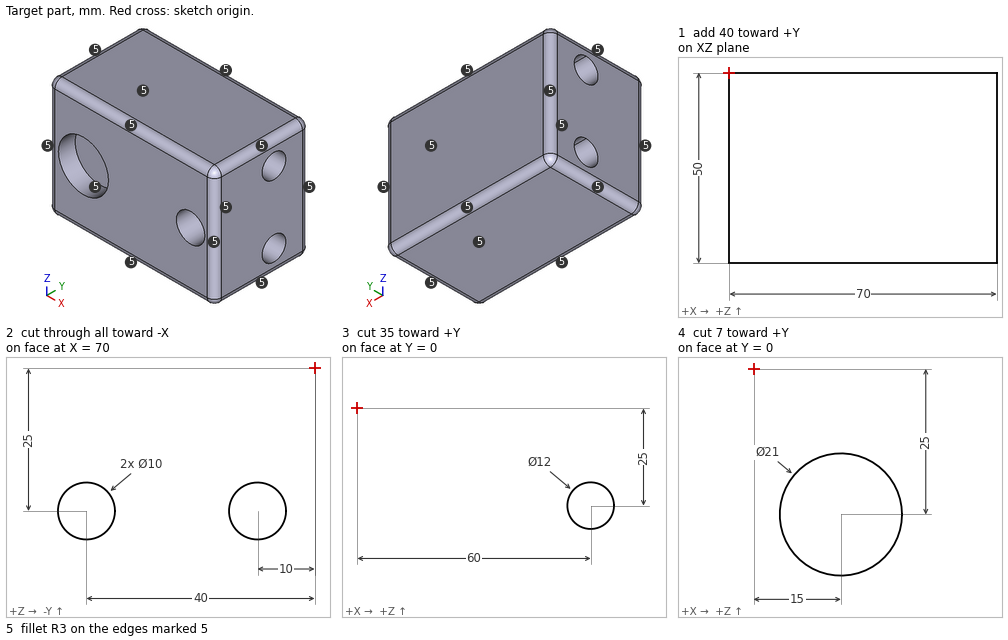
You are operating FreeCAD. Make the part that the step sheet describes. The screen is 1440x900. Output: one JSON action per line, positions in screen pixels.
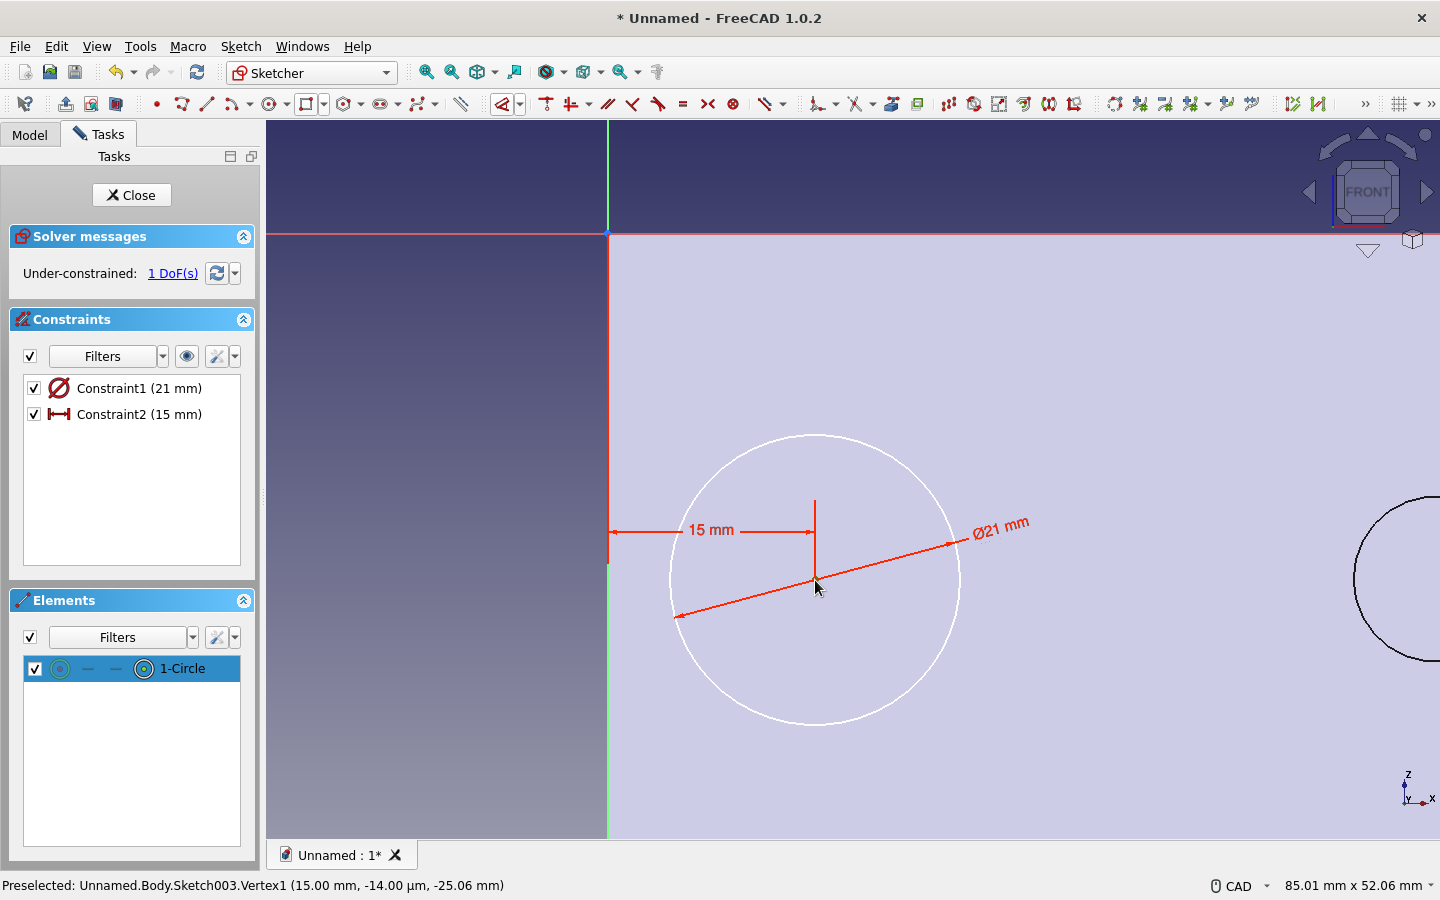
{"action": "key", "text": "i"}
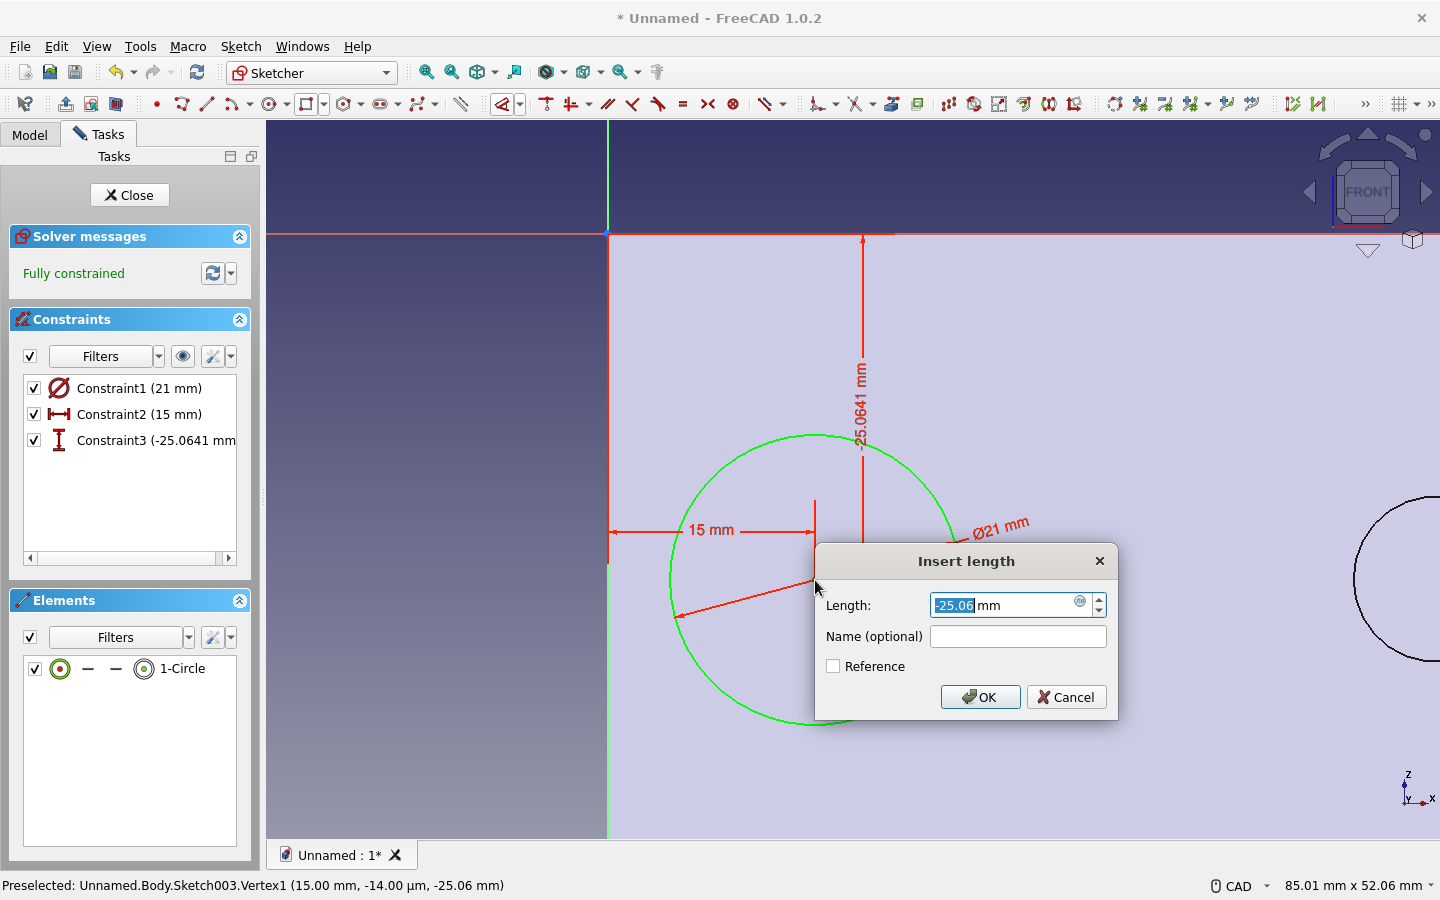
{"action": "type", "text": "-25"}
{"action": "key", "text": "Return"}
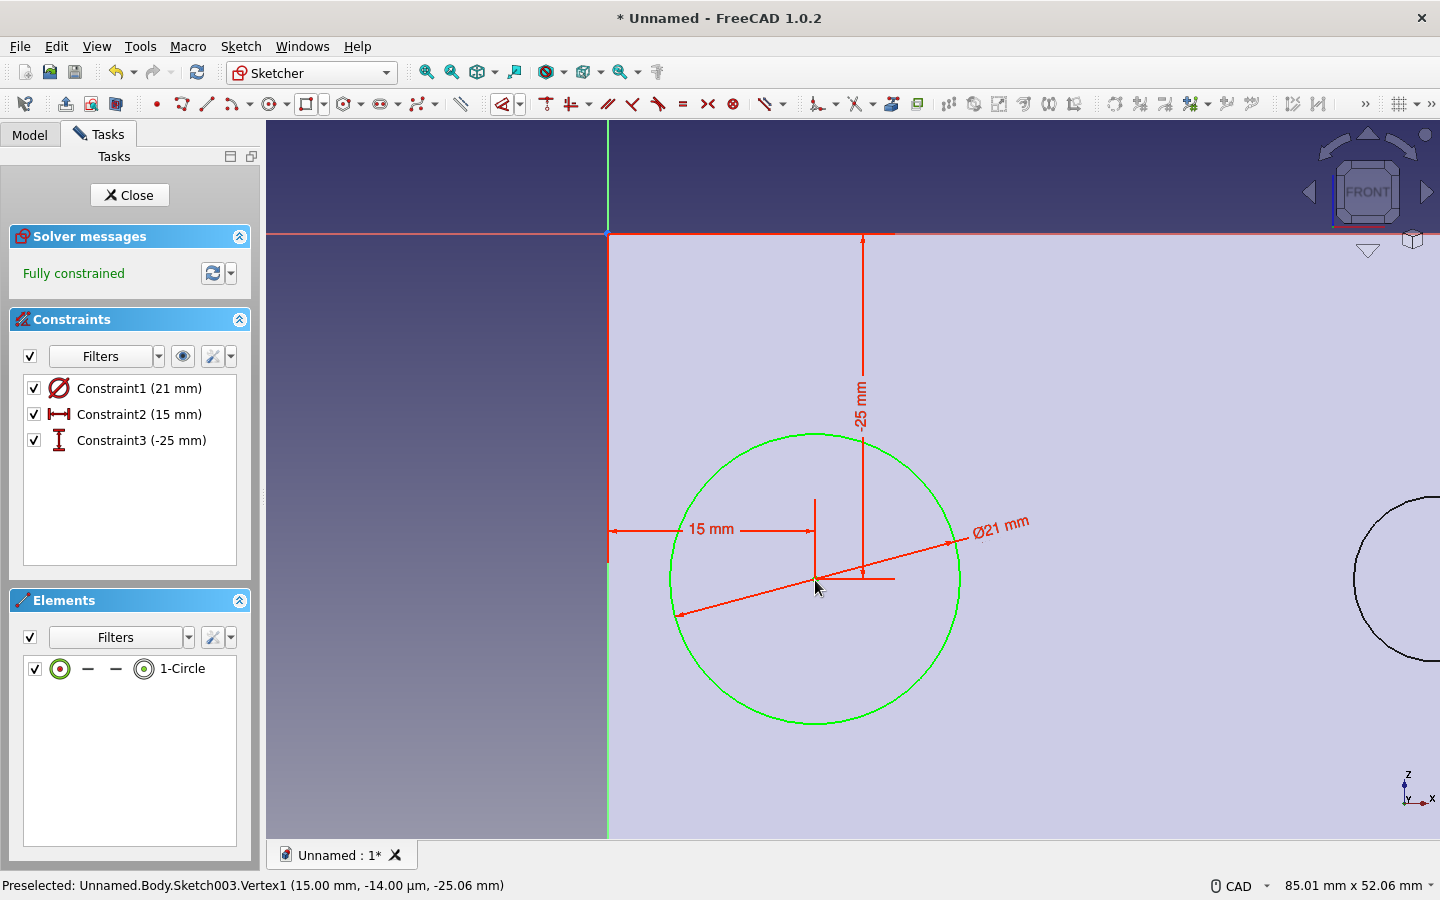
{"action": "left_click", "coordinate": [130, 195]}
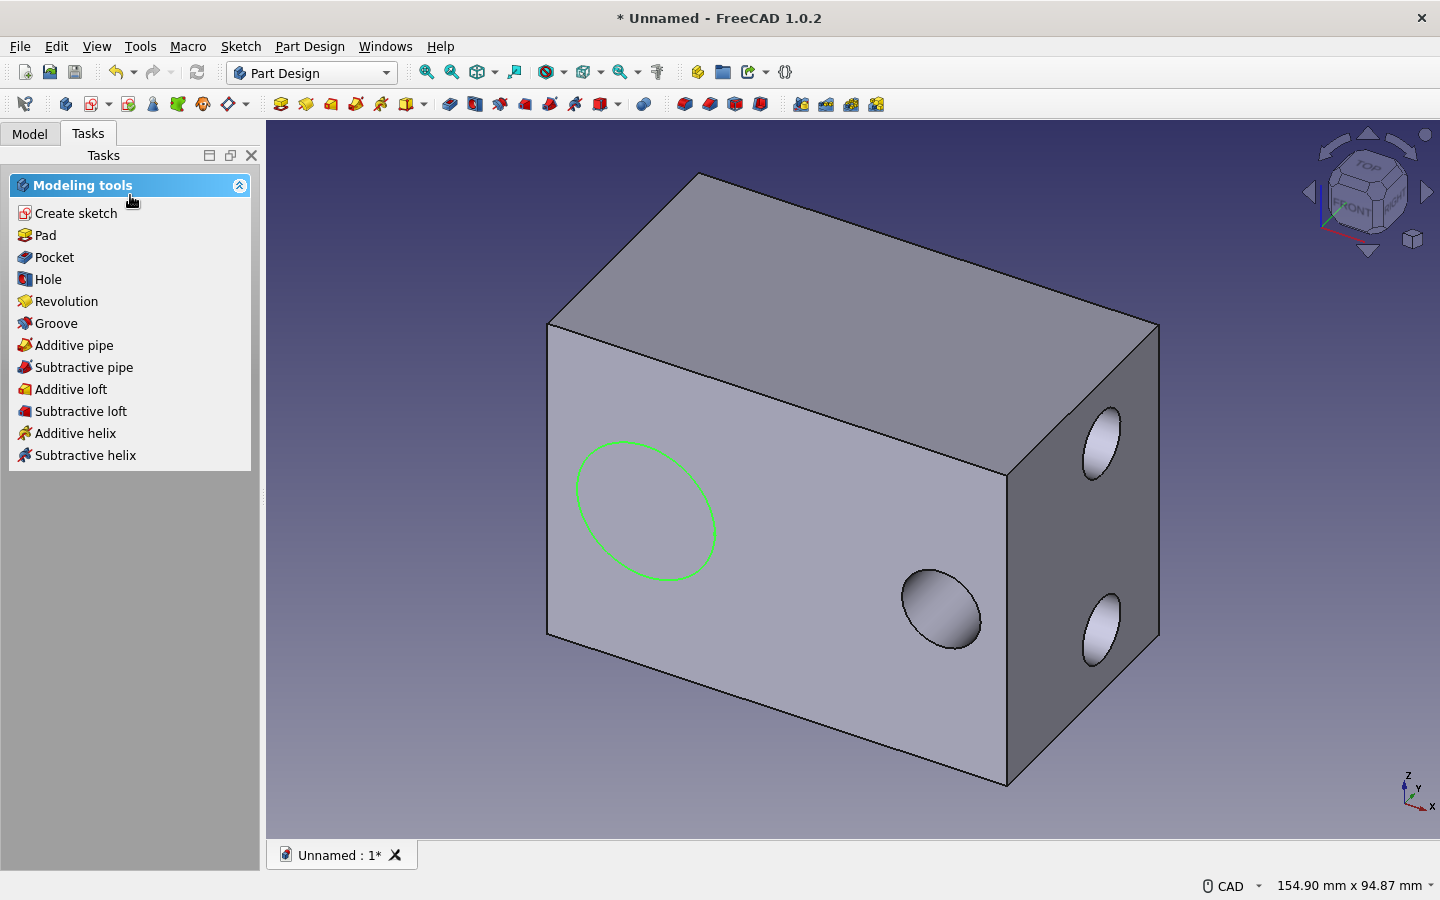
{"action": "left_click", "coordinate": [450, 104]}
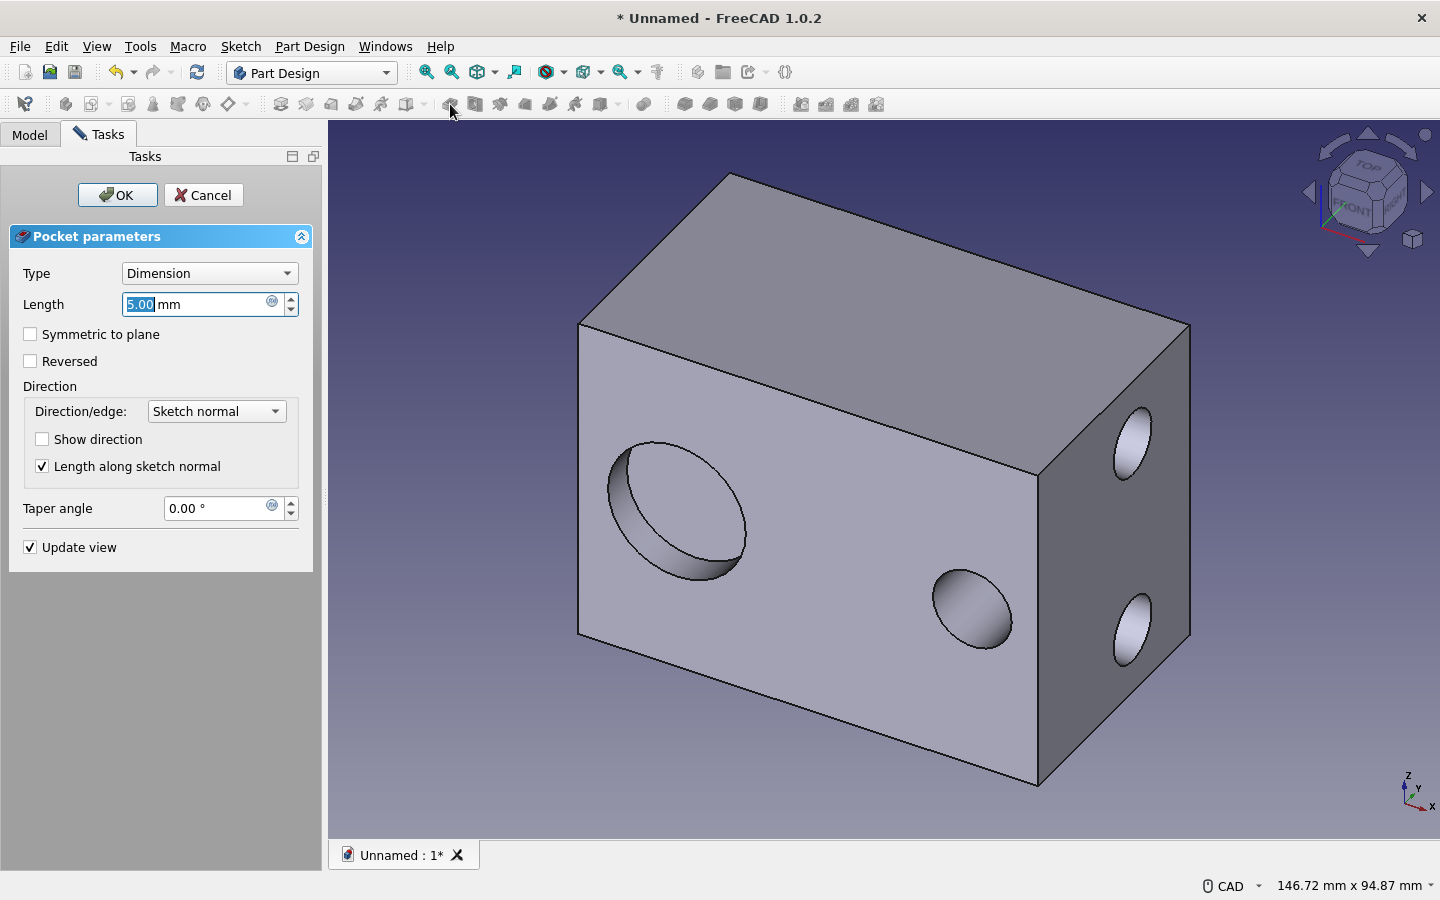
{"action": "type", "text": "7"}
{"action": "key", "text": "Tab"}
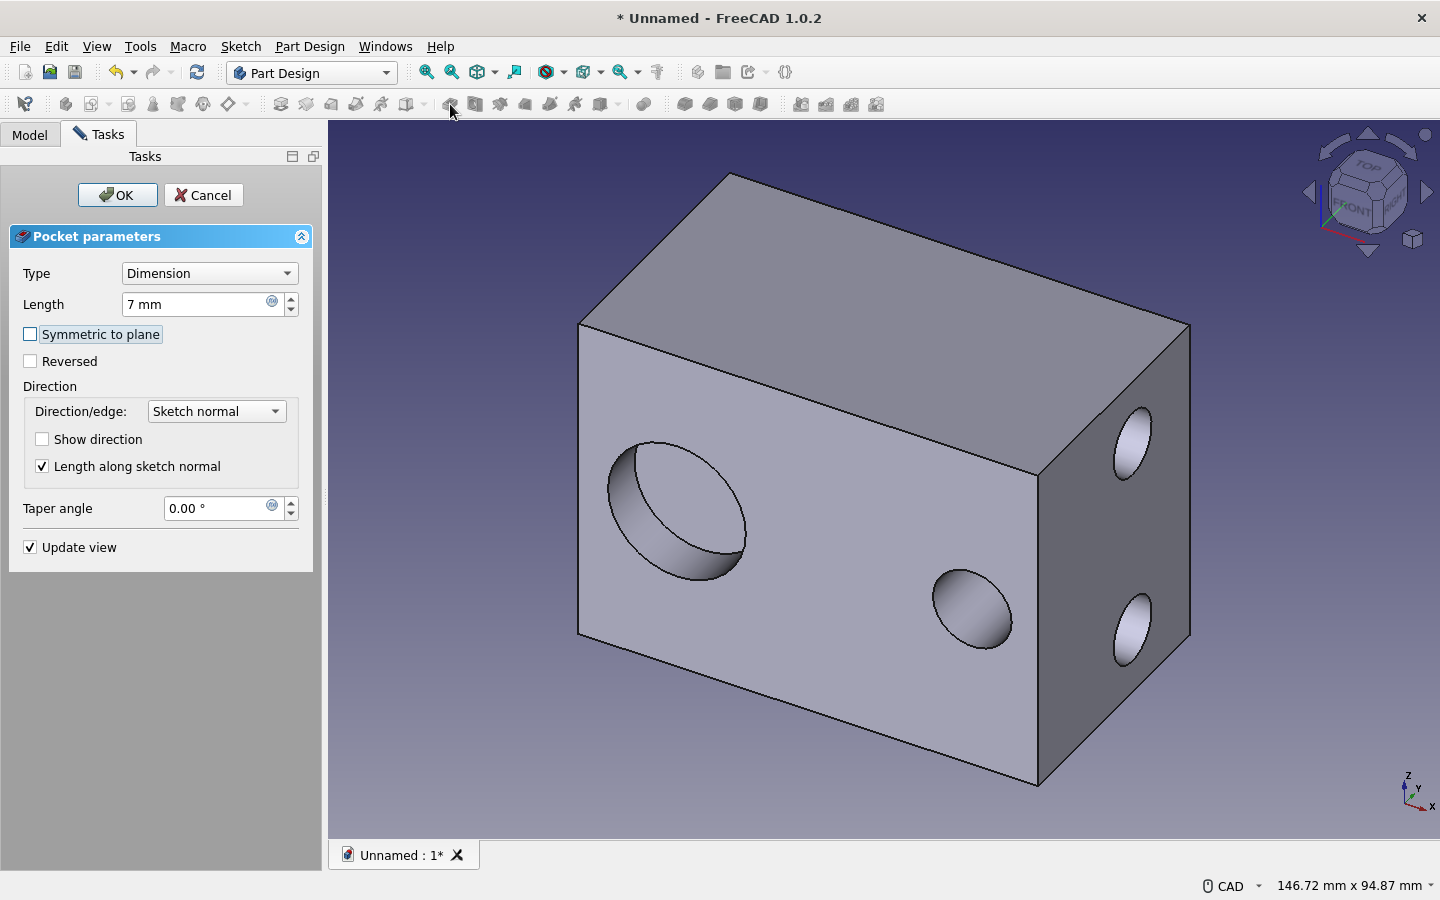
{"action": "left_click", "coordinate": [118, 195]}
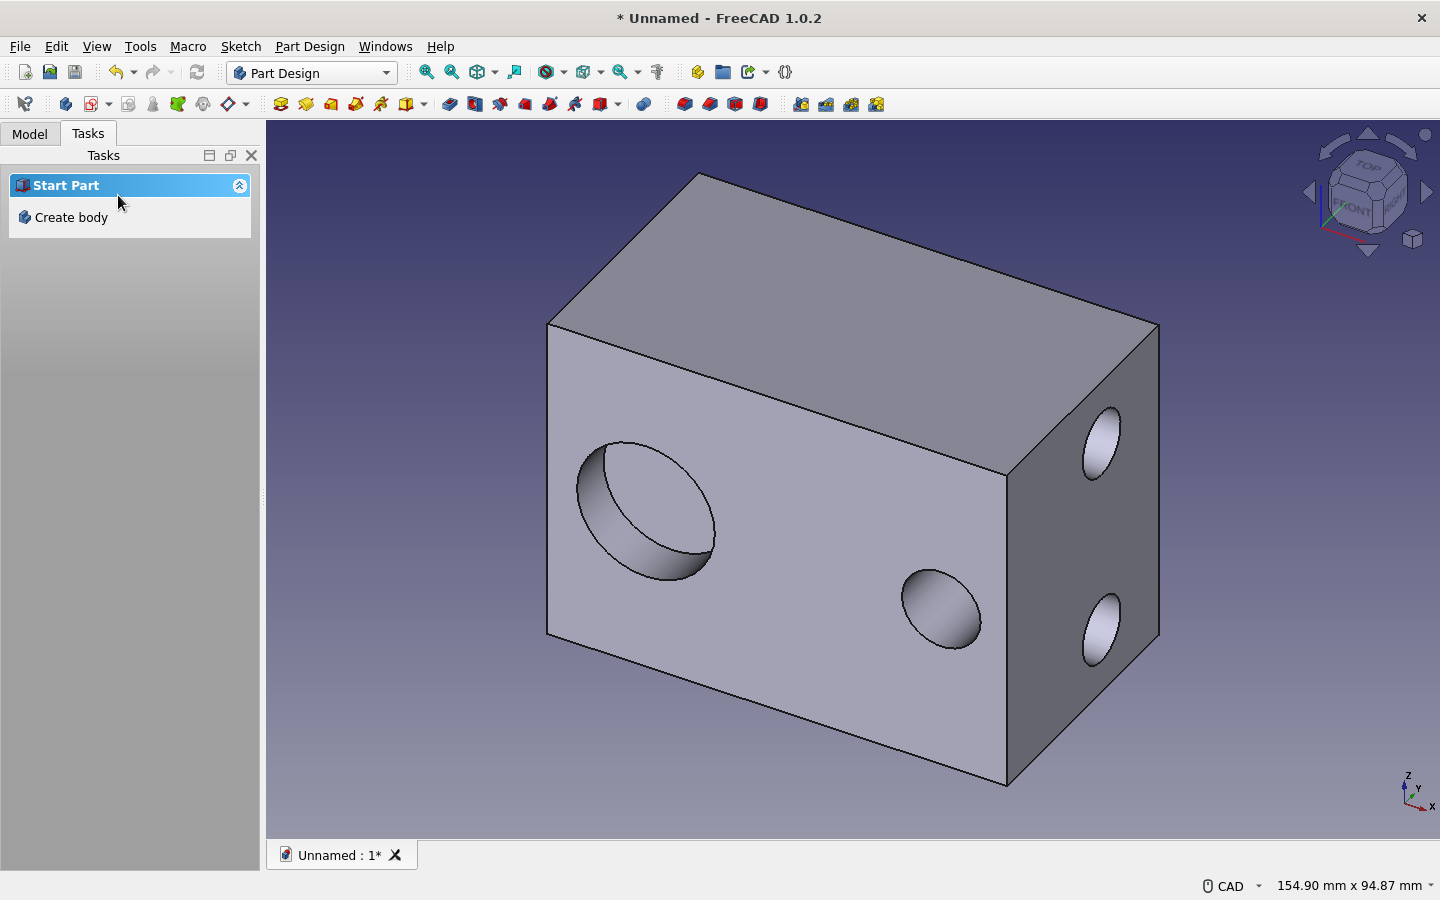
{"action": "left_click", "coordinate": [919, 345]}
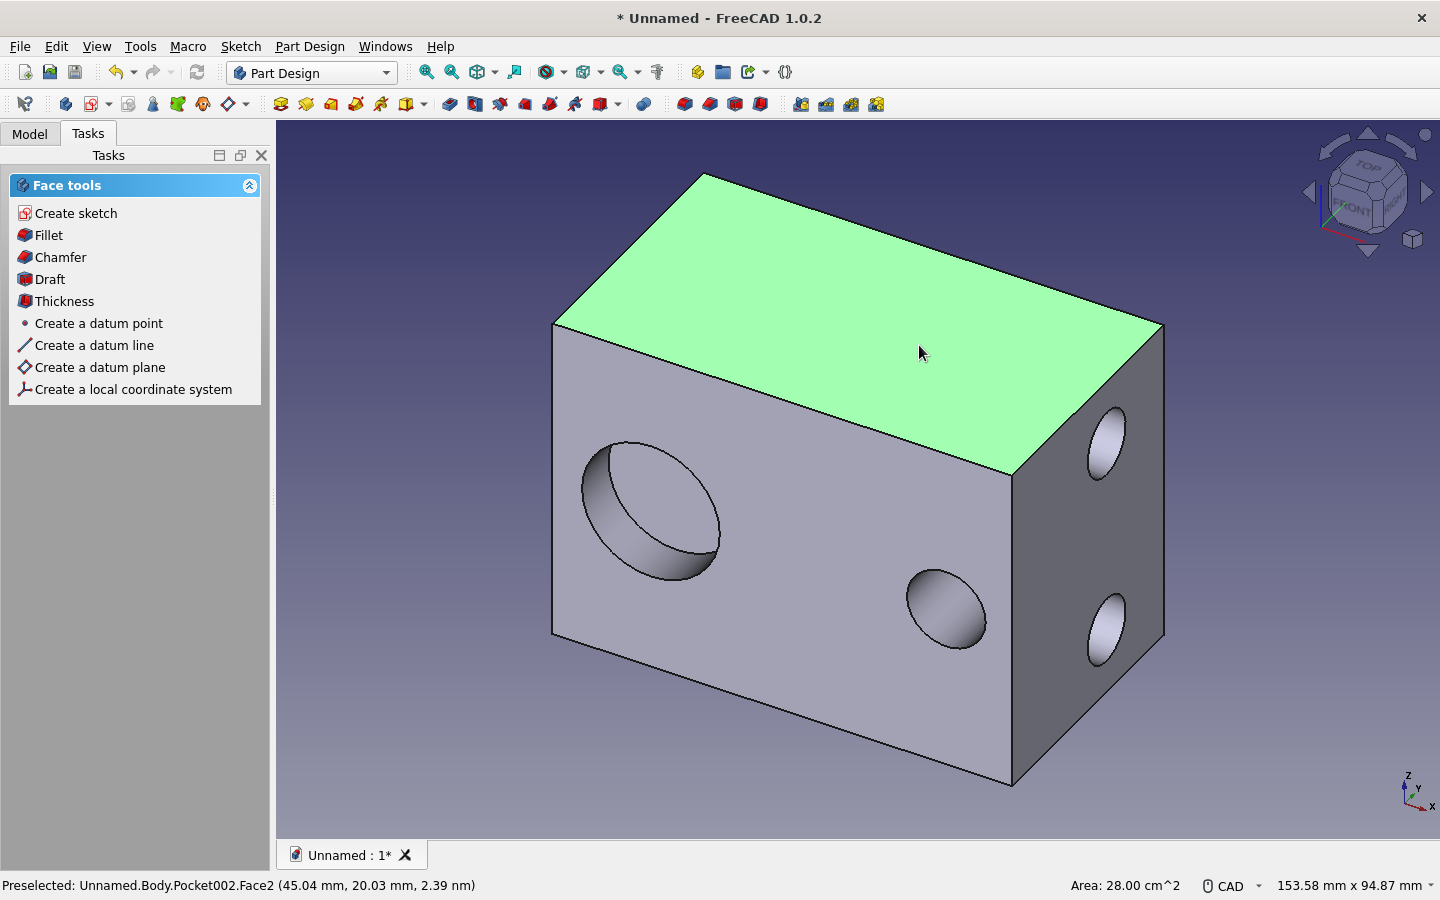
{"action": "left_click", "coordinate": [1012, 630], "text": "ctrl"}